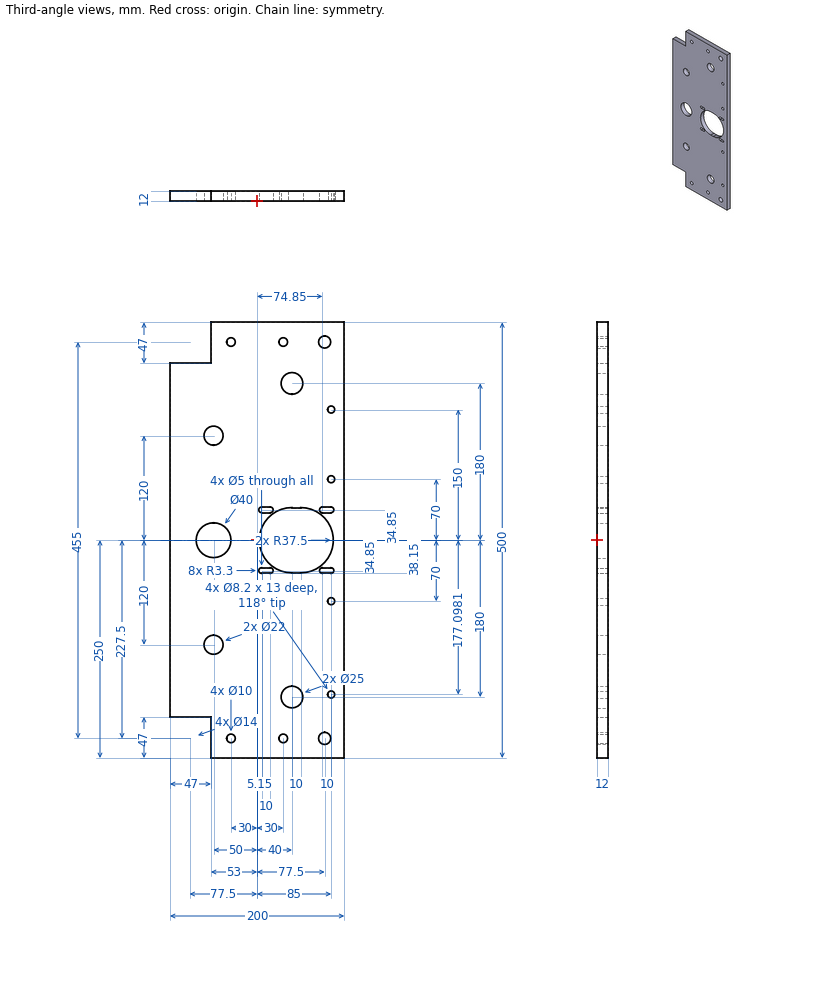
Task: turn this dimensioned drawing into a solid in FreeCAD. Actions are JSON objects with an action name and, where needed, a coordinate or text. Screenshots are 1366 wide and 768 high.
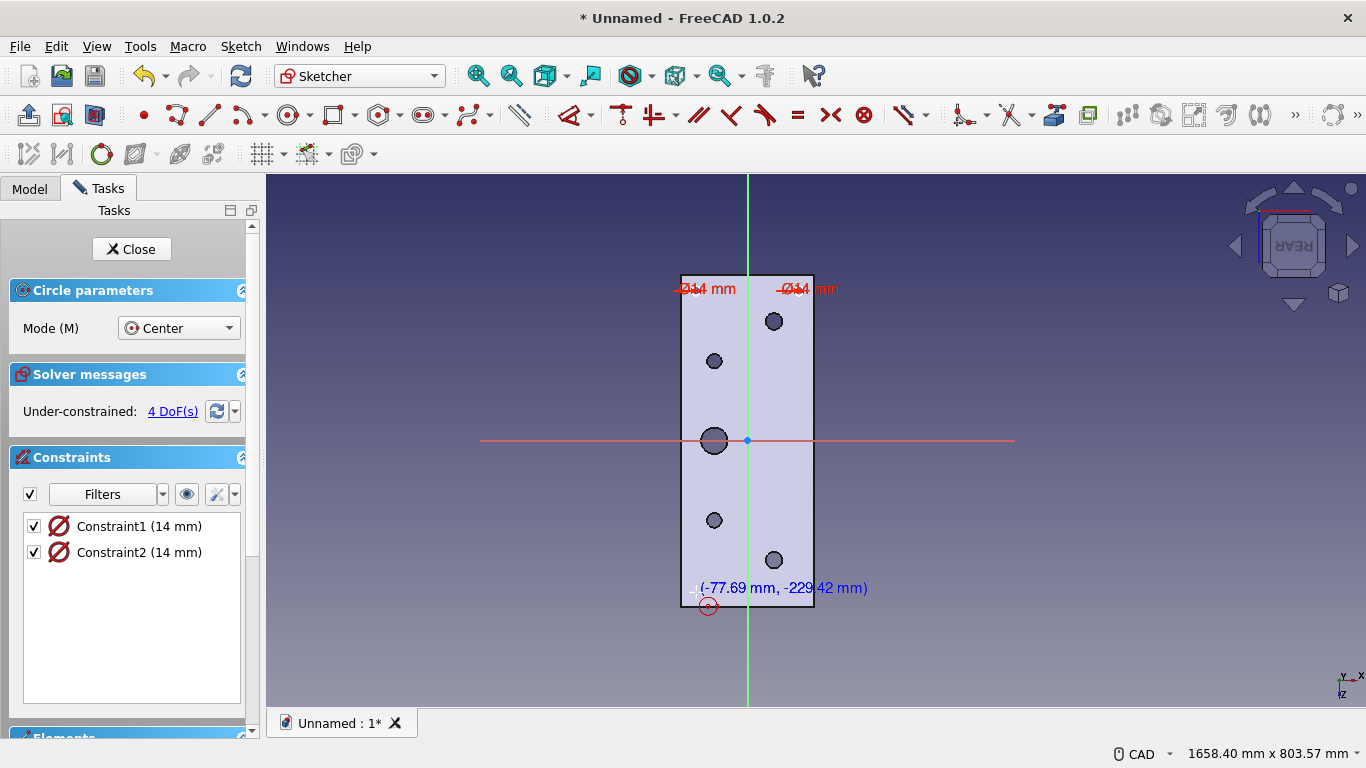
{"action": "left_click", "coordinate": [696, 592]}
{"action": "mouse_move", "coordinate": [699, 588]}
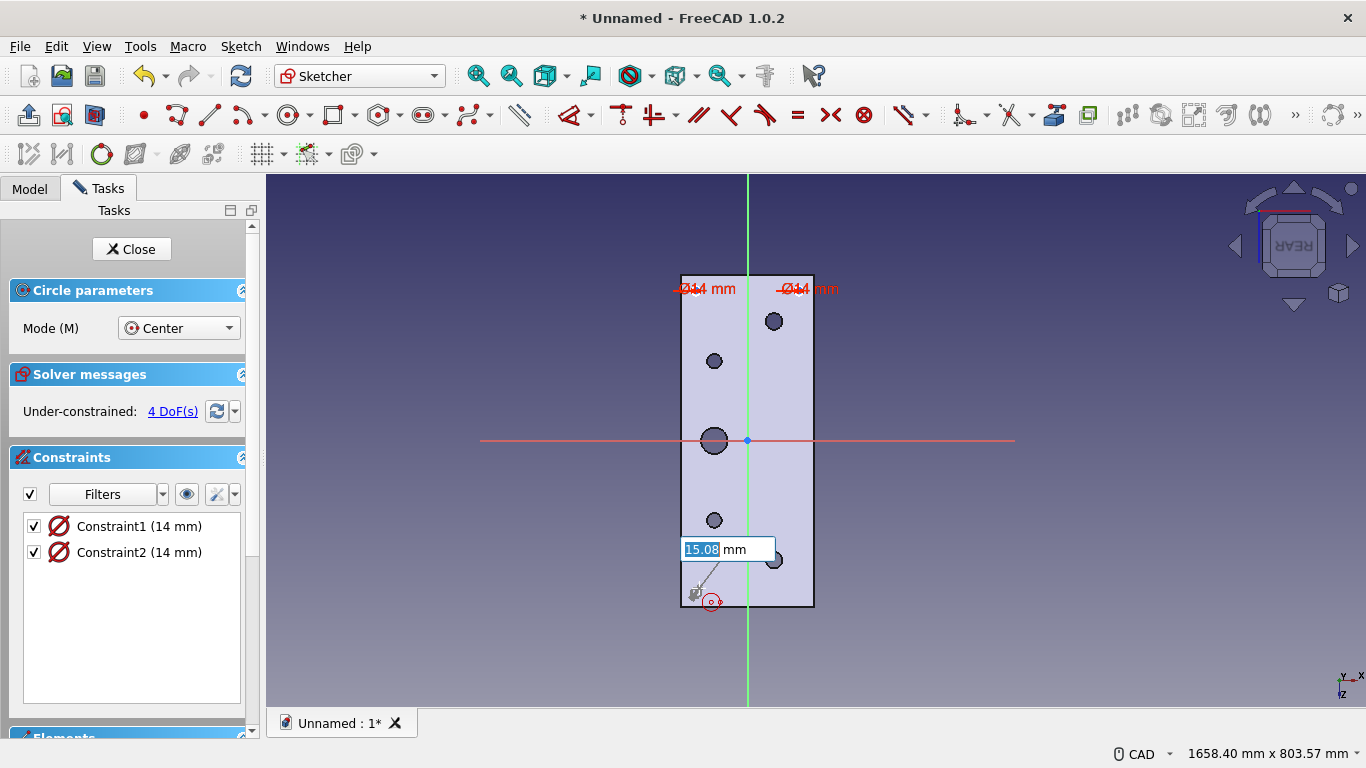
{"action": "type", "text": "14"}
{"action": "key", "text": "Return"}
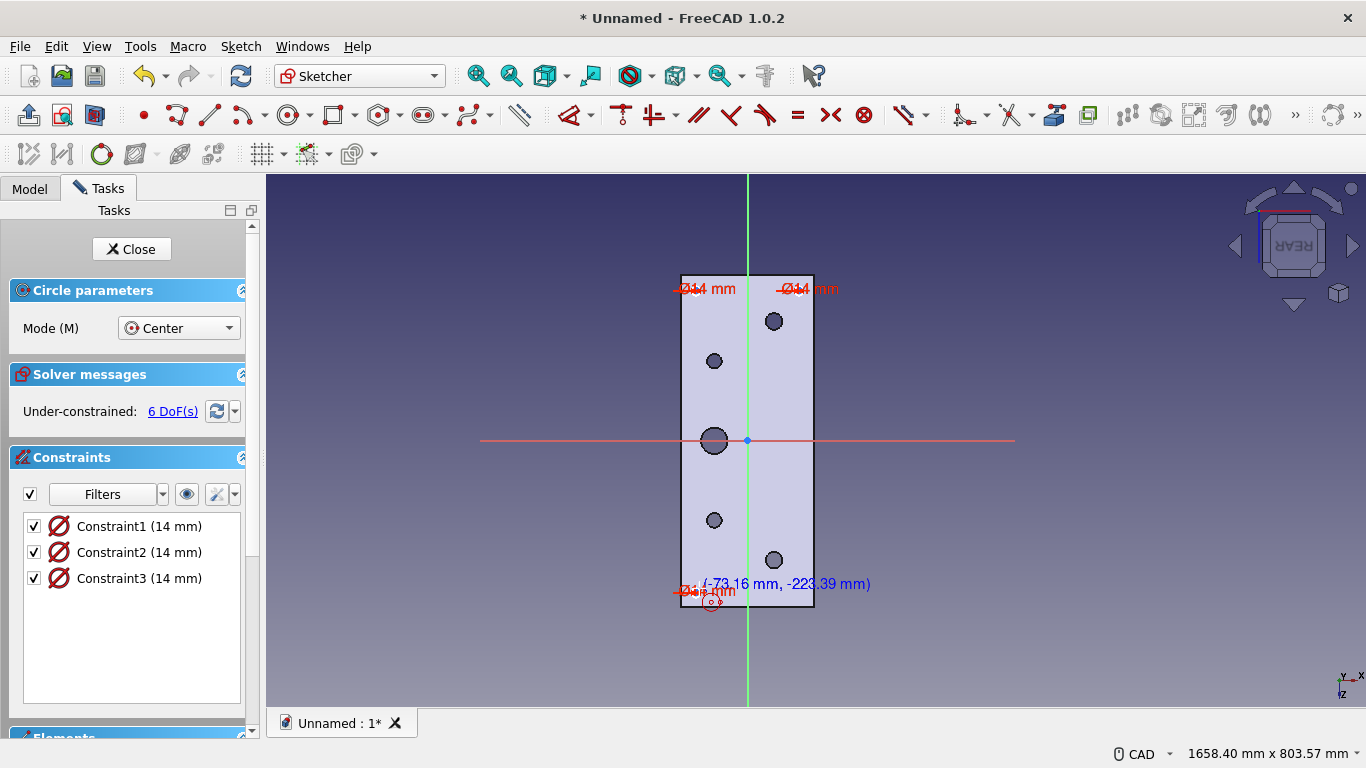
{"action": "scroll", "coordinate": [799, 592], "scroll_direction": "up", "scroll_amount": 8}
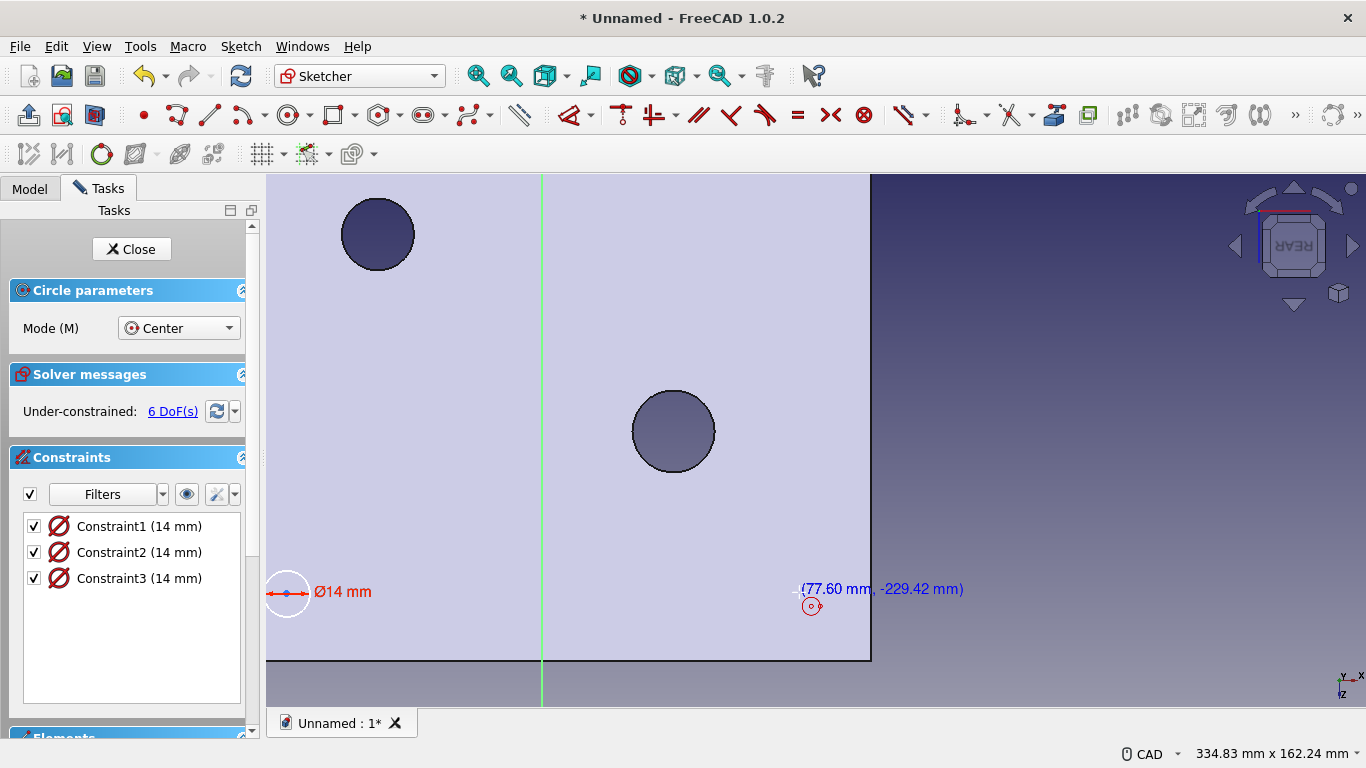
{"action": "scroll", "coordinate": [799, 592], "scroll_direction": "down", "scroll_amount": 8}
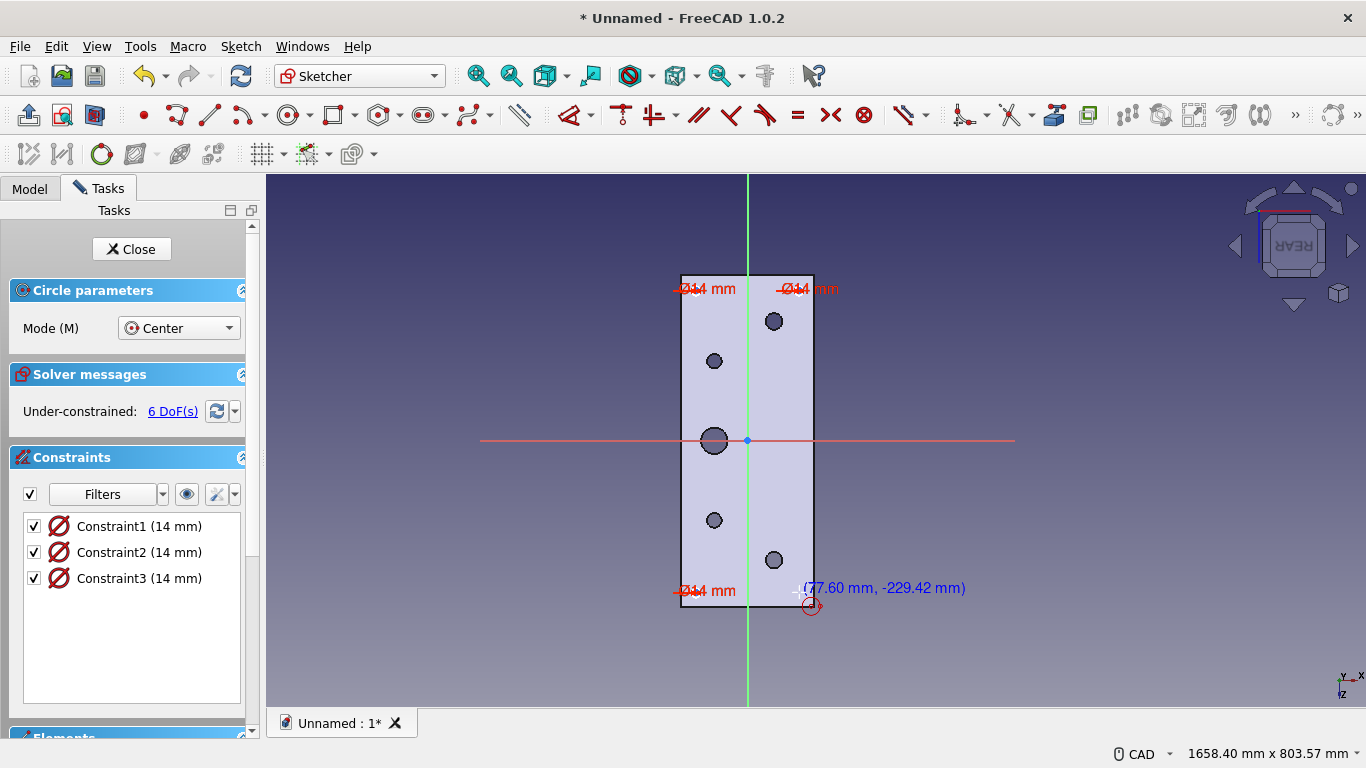
{"action": "left_click", "coordinate": [799, 592]}
{"action": "mouse_move", "coordinate": [802, 588]}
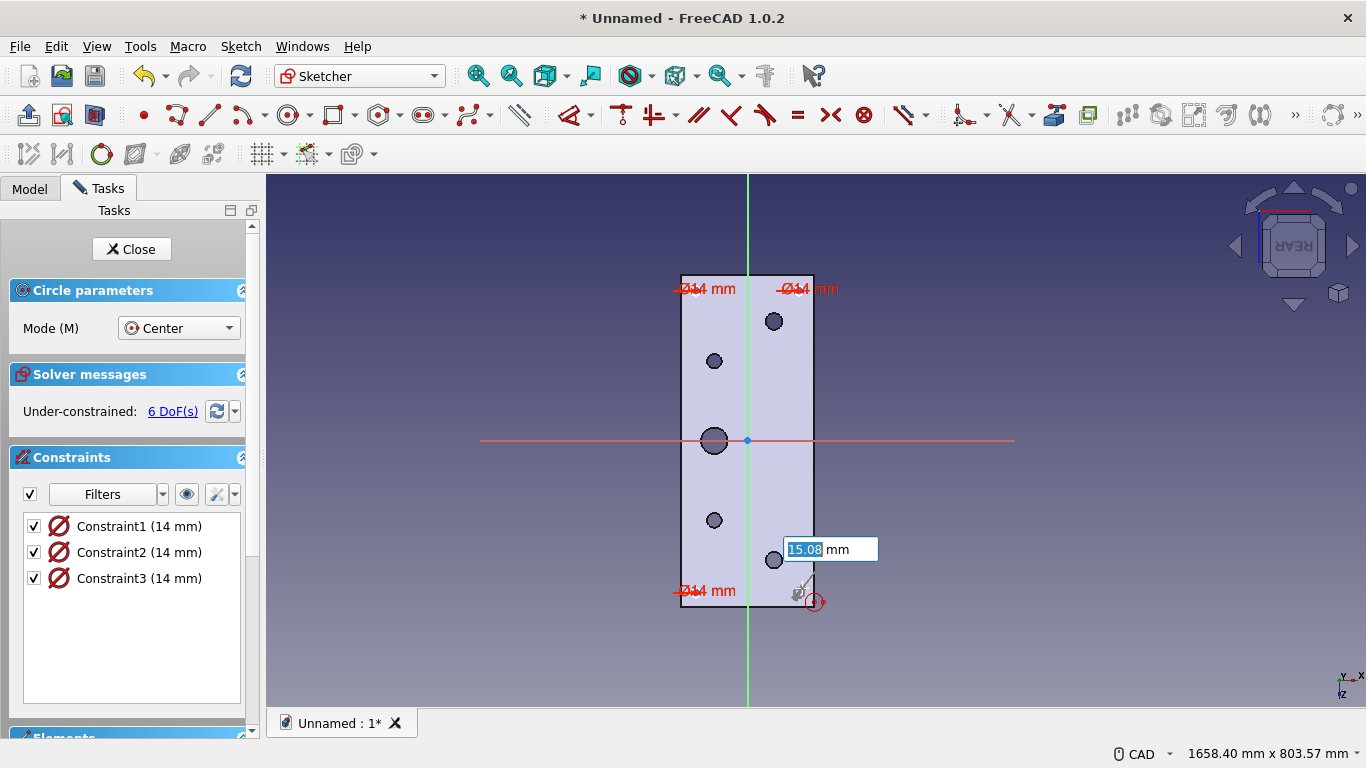
{"action": "type", "text": "14"}
{"action": "key", "text": "Return"}
{"action": "key", "text": "Escape"}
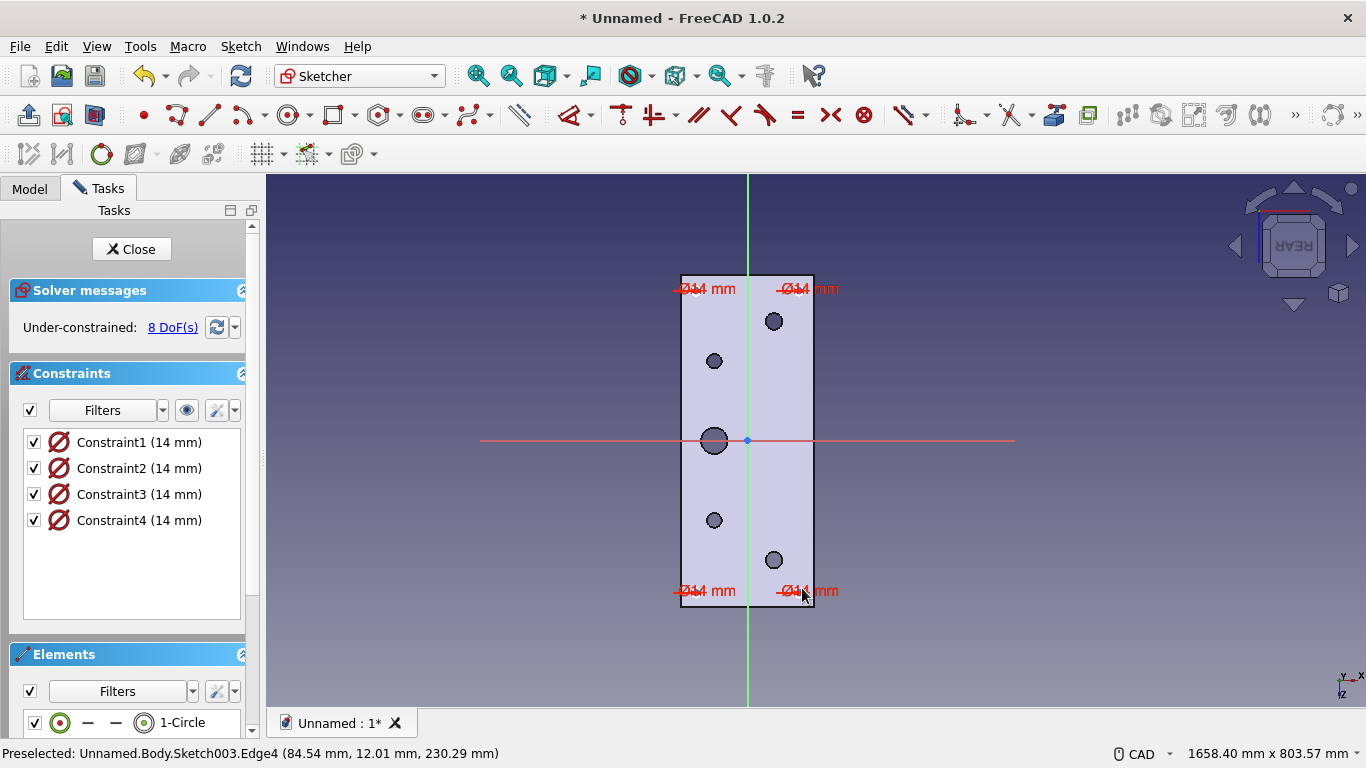
{"action": "left_click", "coordinate": [696, 291]}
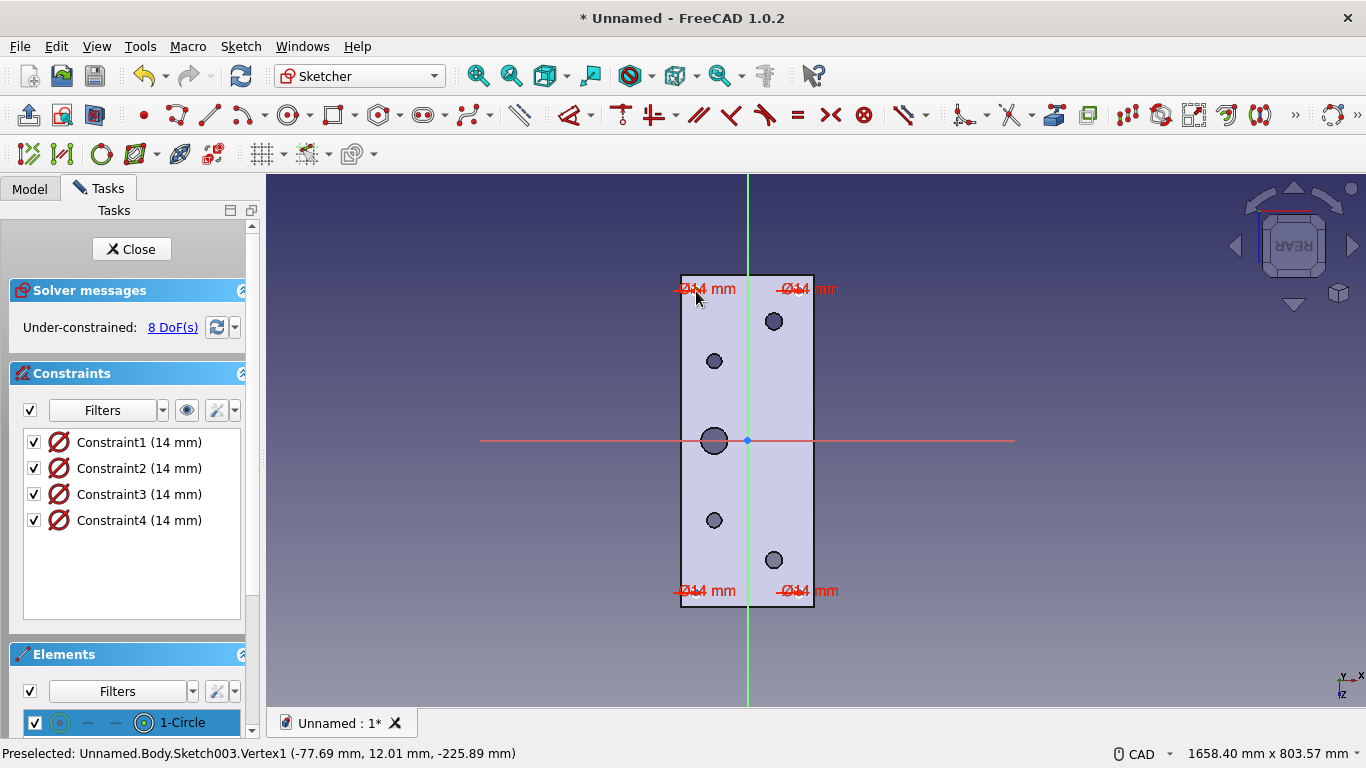
{"action": "left_click", "coordinate": [799, 291]}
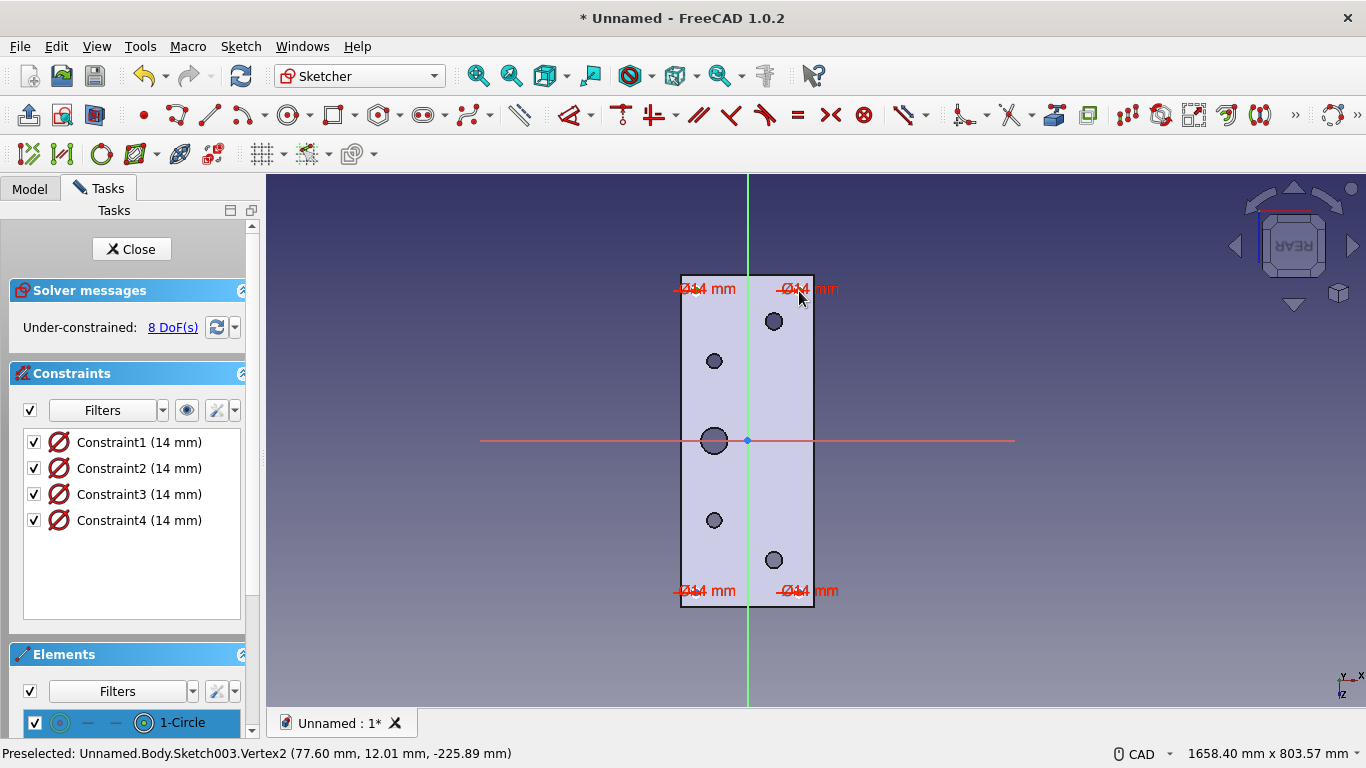
{"action": "key", "text": "h"}